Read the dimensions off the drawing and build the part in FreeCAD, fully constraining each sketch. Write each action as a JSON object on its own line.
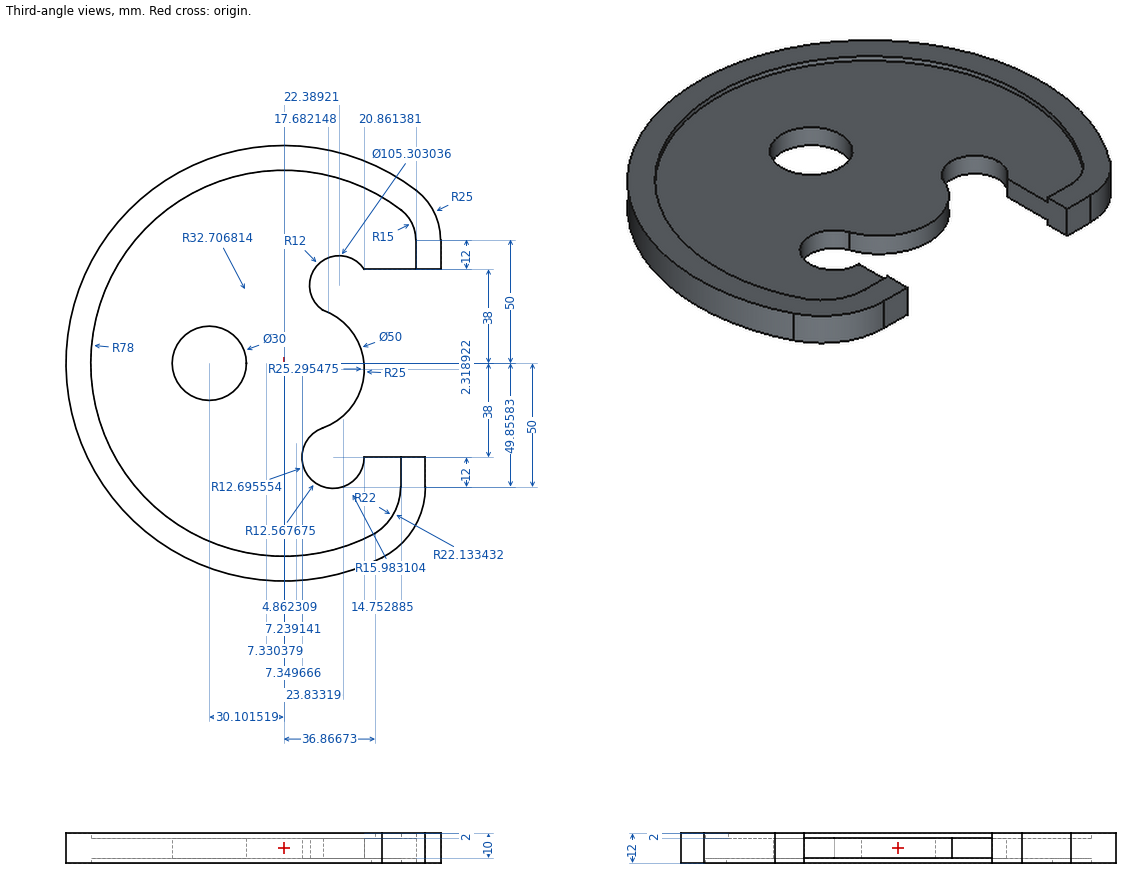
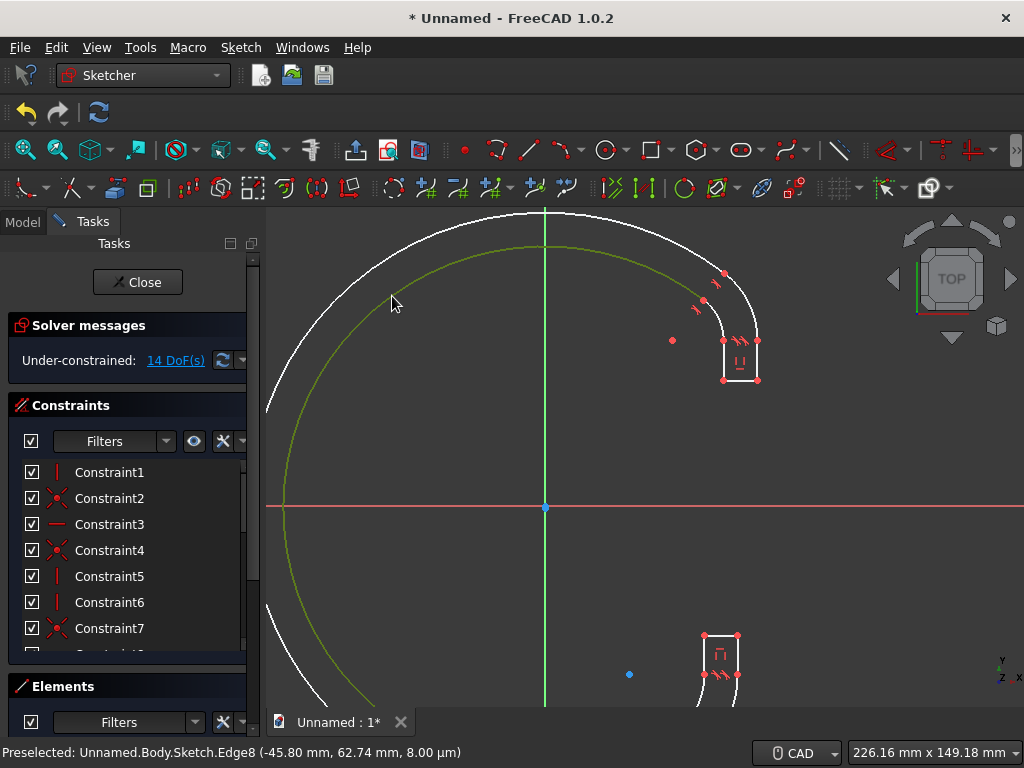
{"action": "left_click", "coordinate": [372, 269]}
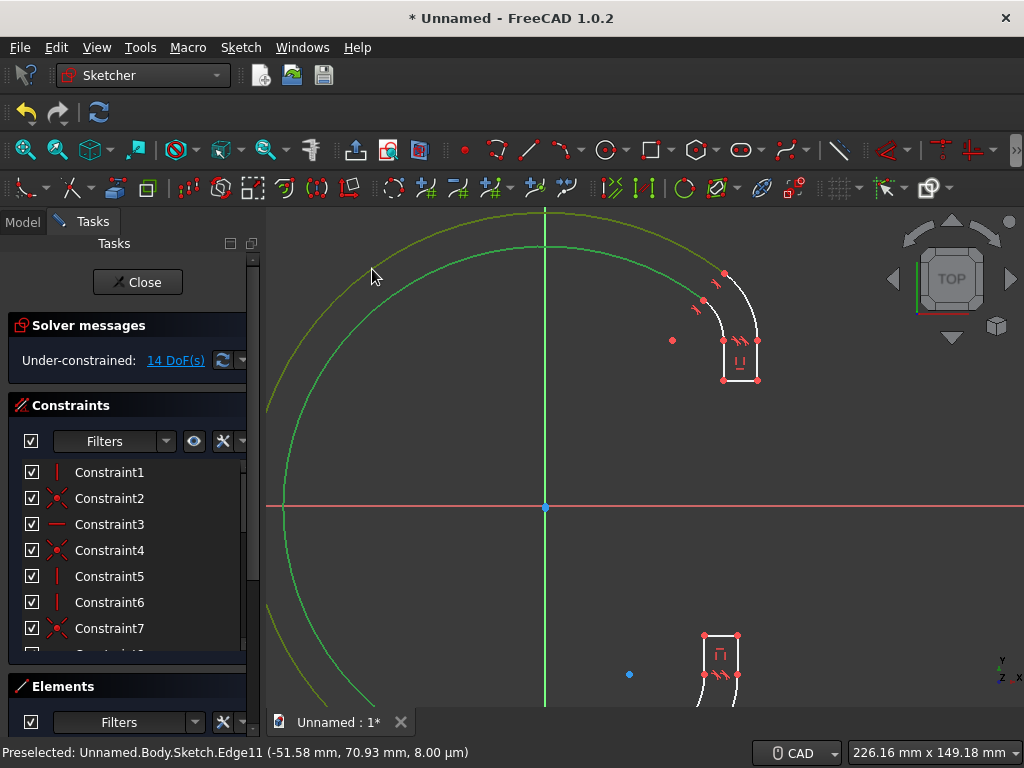
{"action": "left_click", "coordinate": [942, 150]}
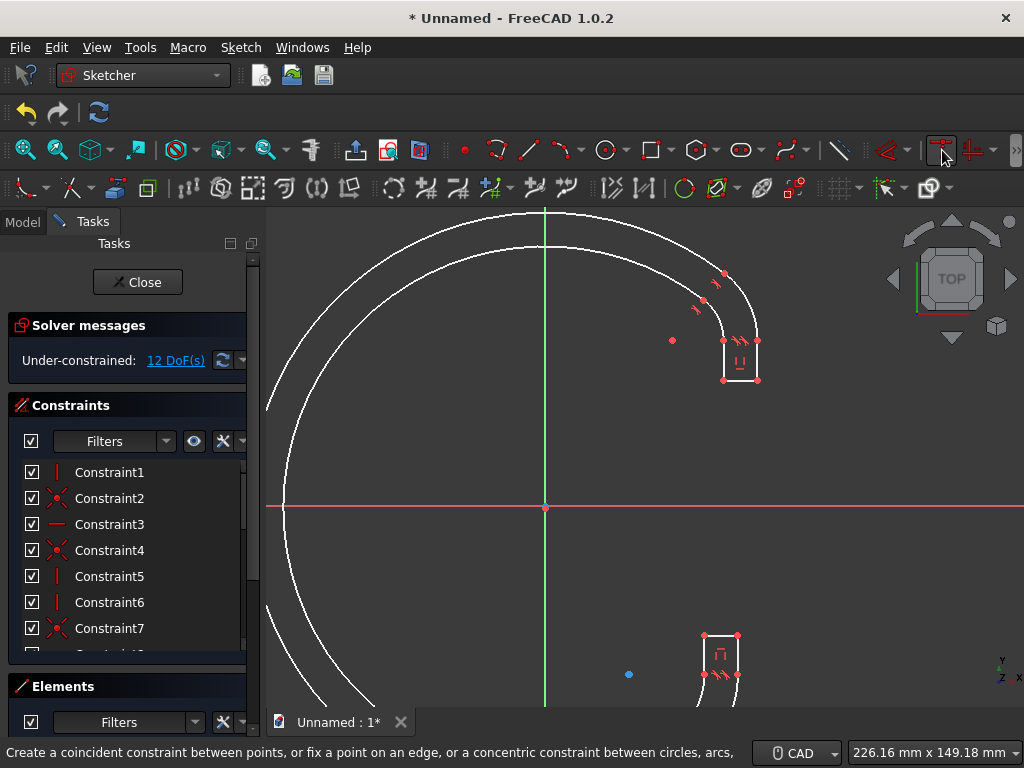
{"action": "scroll", "coordinate": [723, 327], "scroll_direction": "down", "scroll_amount": 2}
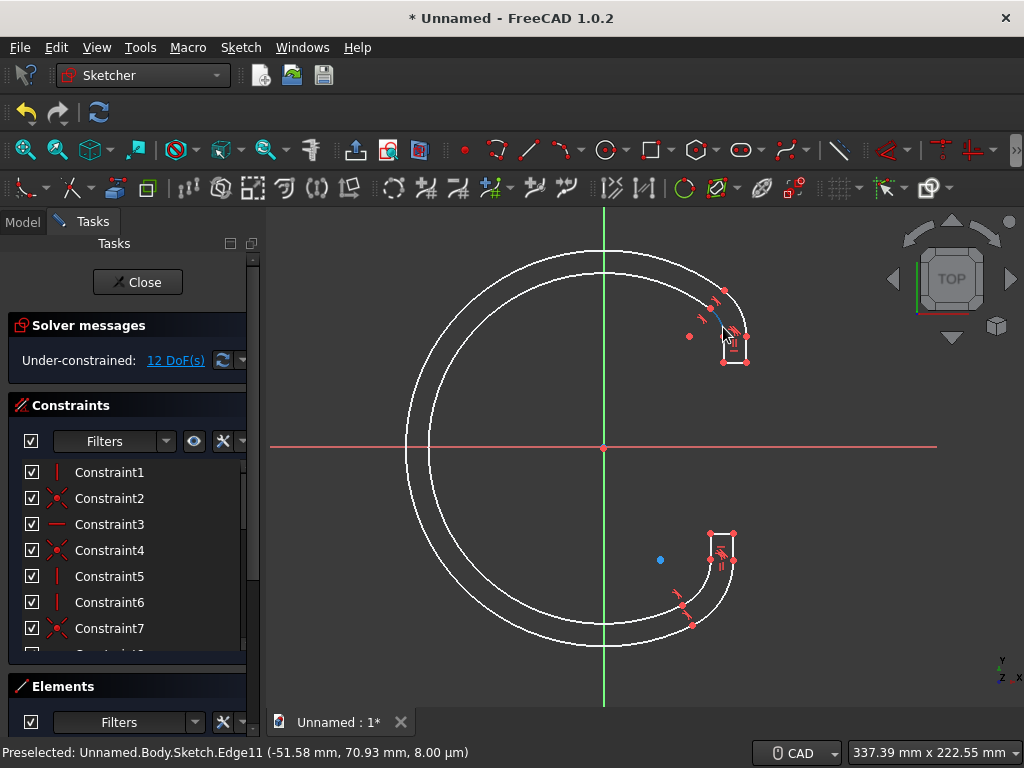
{"action": "left_click", "coordinate": [696, 595]}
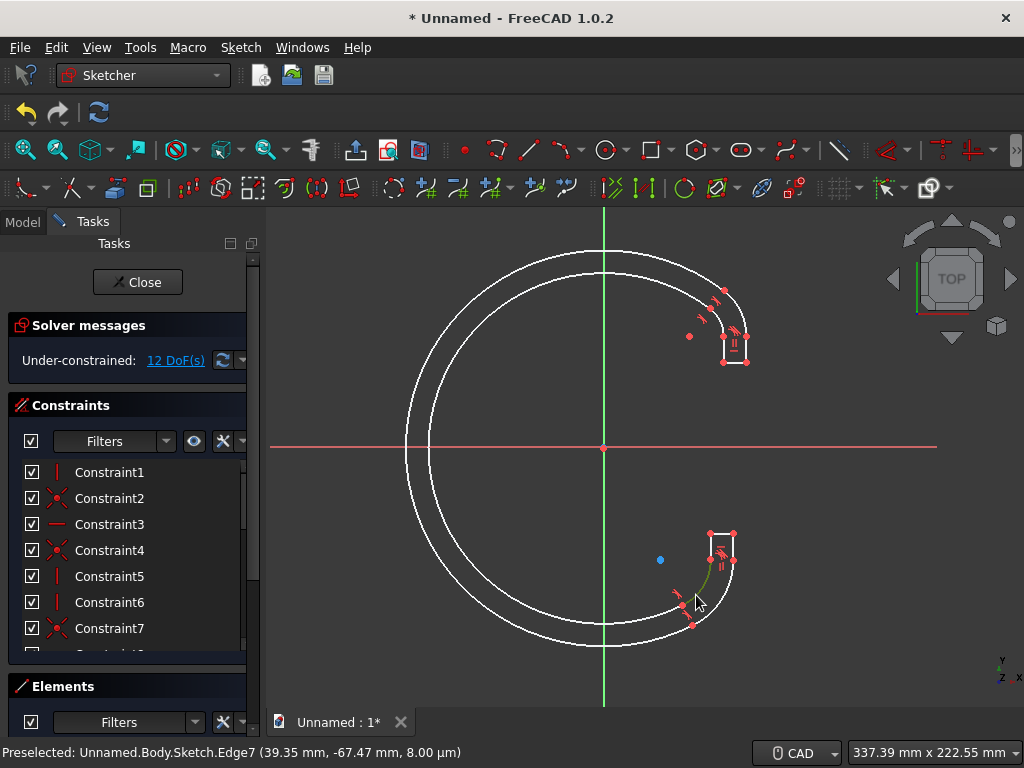
{"action": "left_click", "coordinate": [712, 611]}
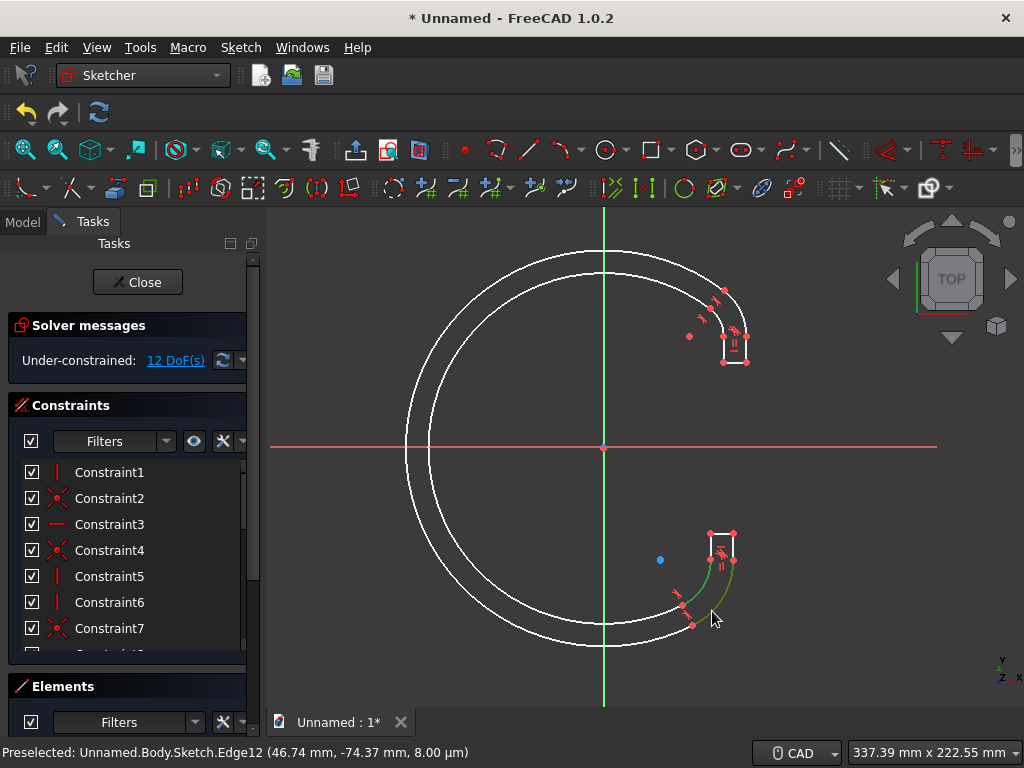
{"action": "key", "text": "c"}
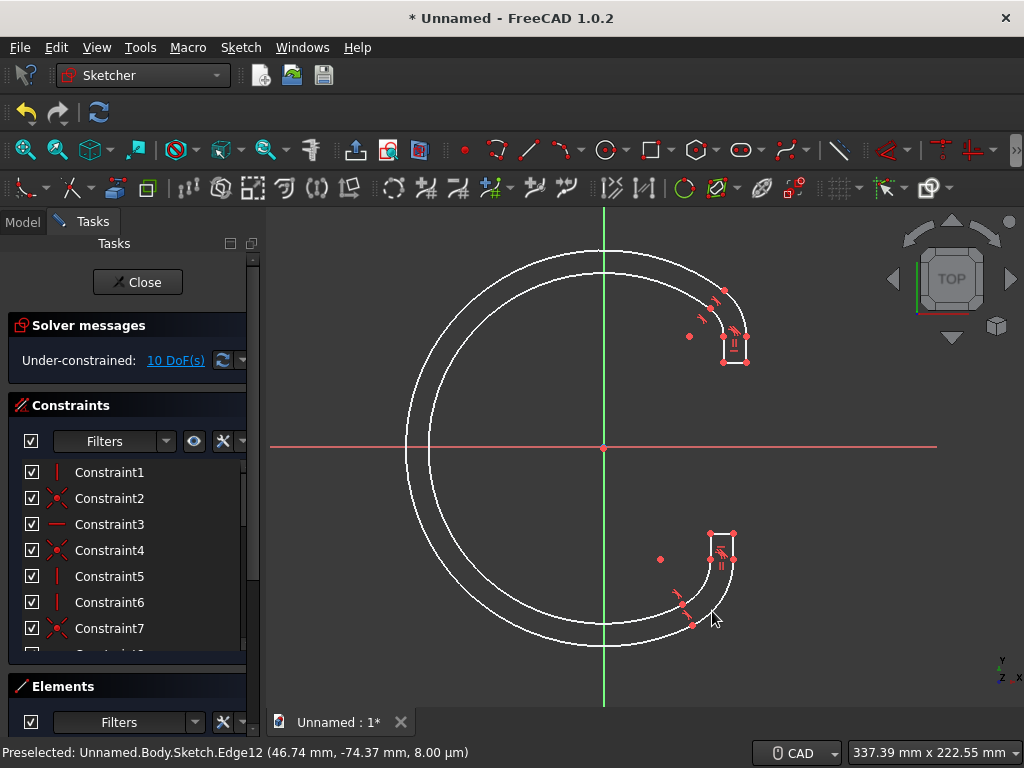
{"action": "left_click_drag", "start_coordinate": [594, 437], "coordinate": [614, 458]}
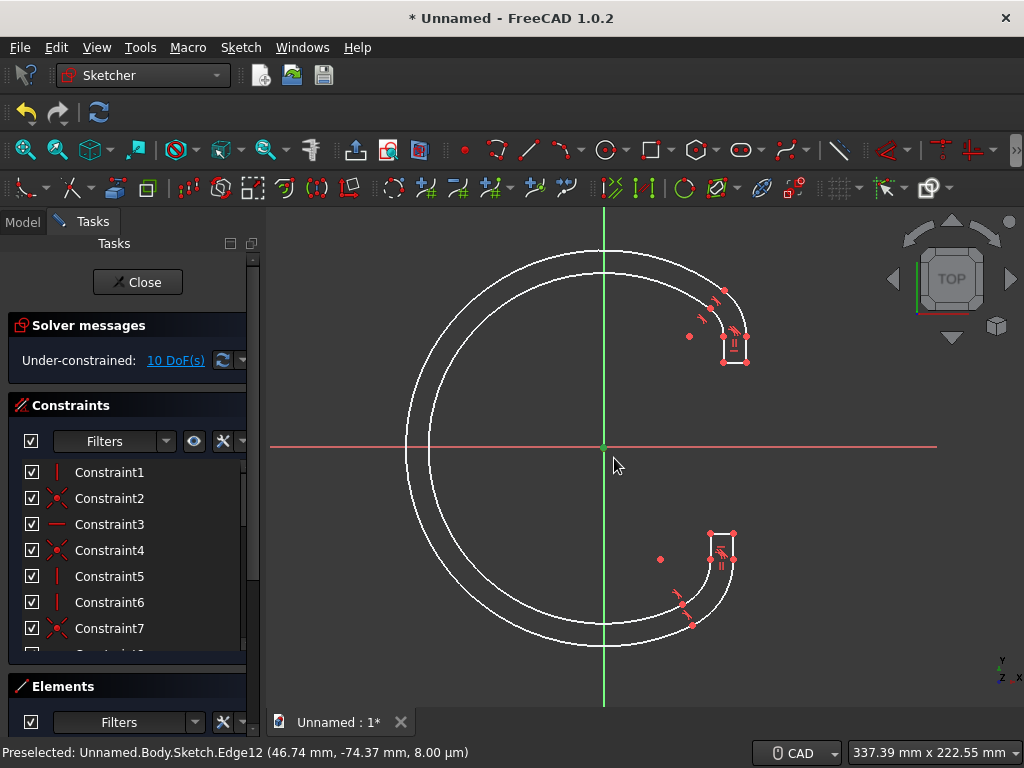
{"action": "key", "text": "c"}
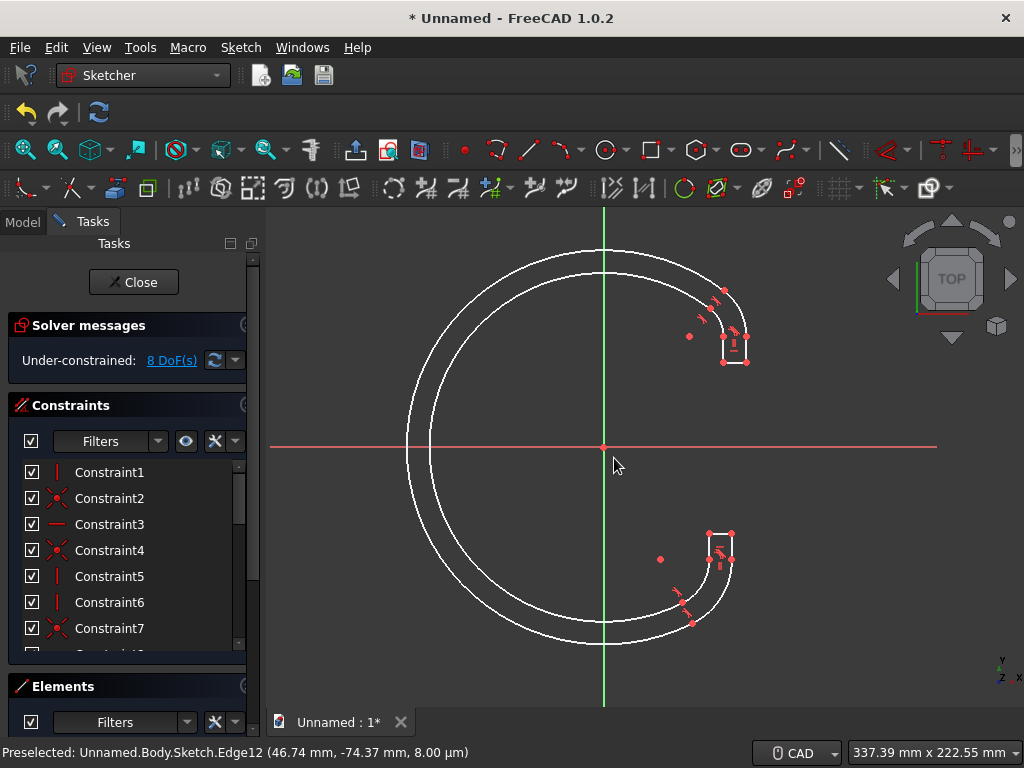
{"action": "key", "text": "d"}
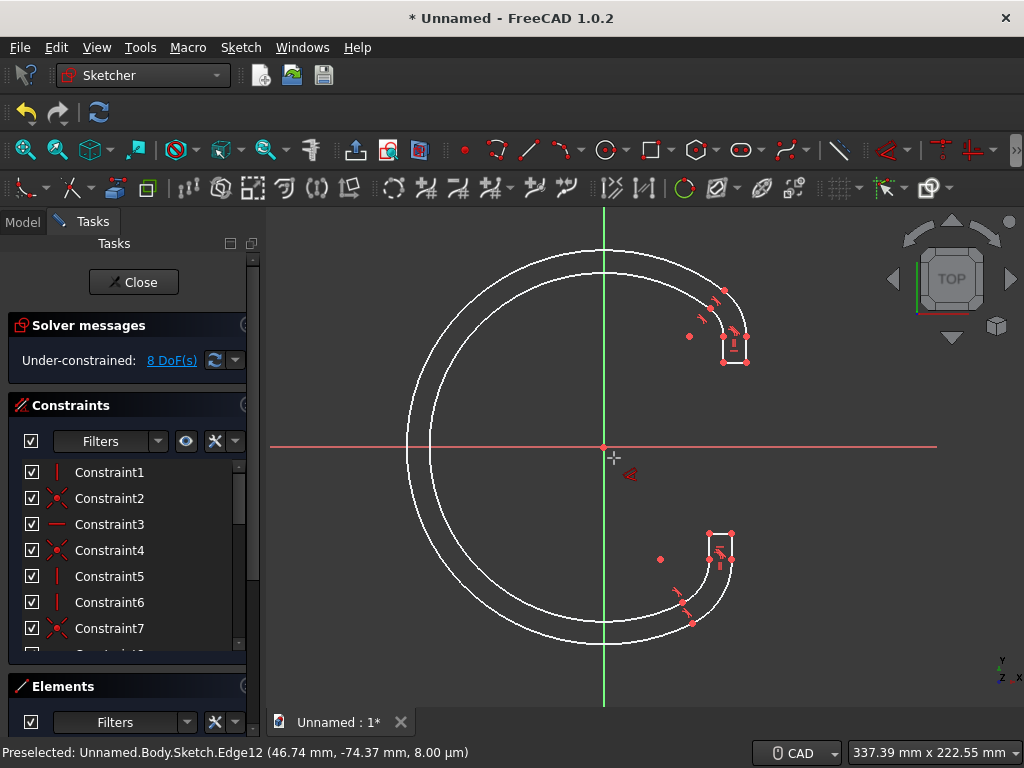
{"action": "left_click", "coordinate": [696, 594]}
{"action": "left_click", "coordinate": [717, 502]}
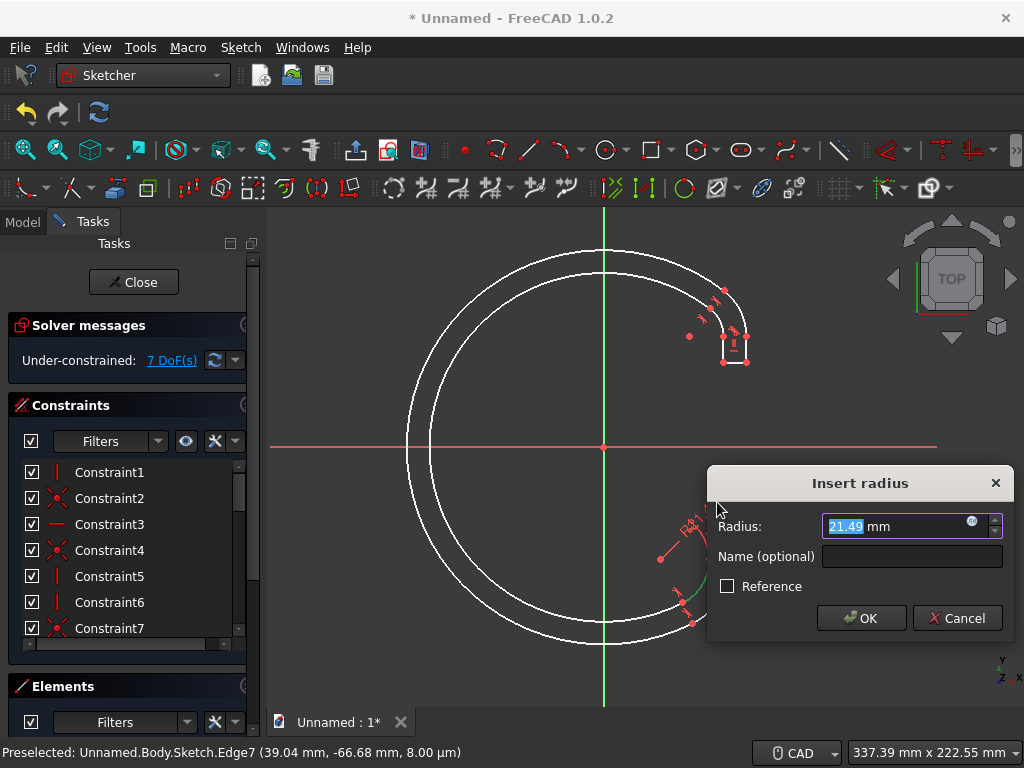
{"action": "type", "text": "22"}
{"action": "key", "text": "Return"}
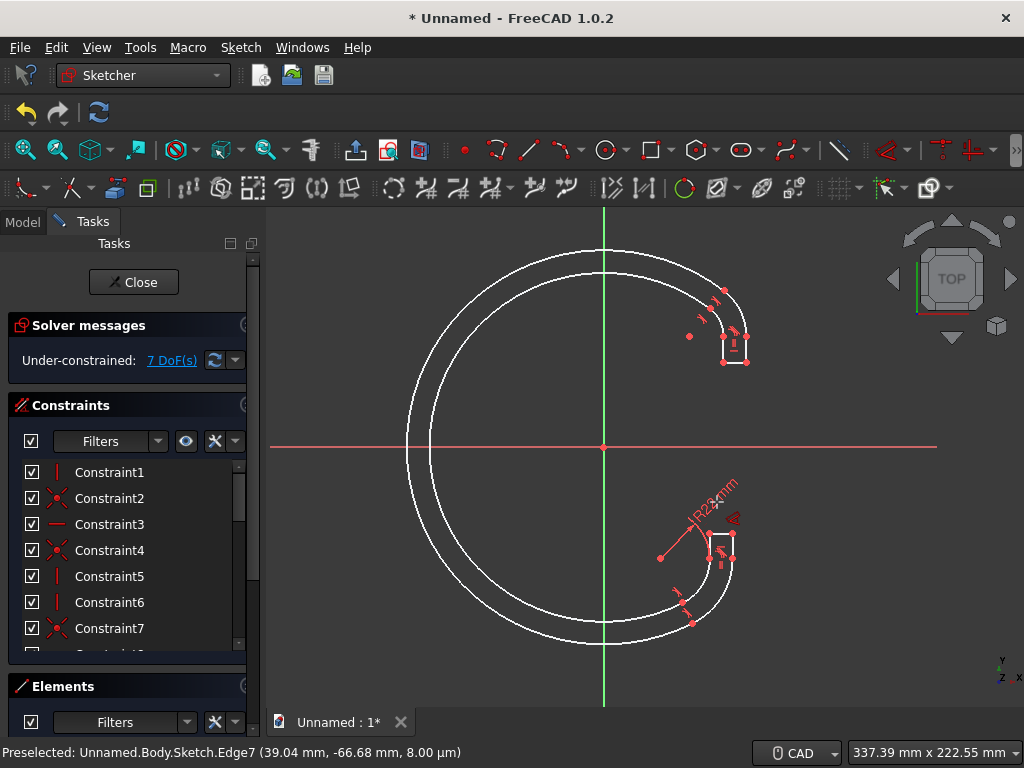
{"action": "left_click", "coordinate": [502, 306]}
{"action": "left_click", "coordinate": [771, 327]}